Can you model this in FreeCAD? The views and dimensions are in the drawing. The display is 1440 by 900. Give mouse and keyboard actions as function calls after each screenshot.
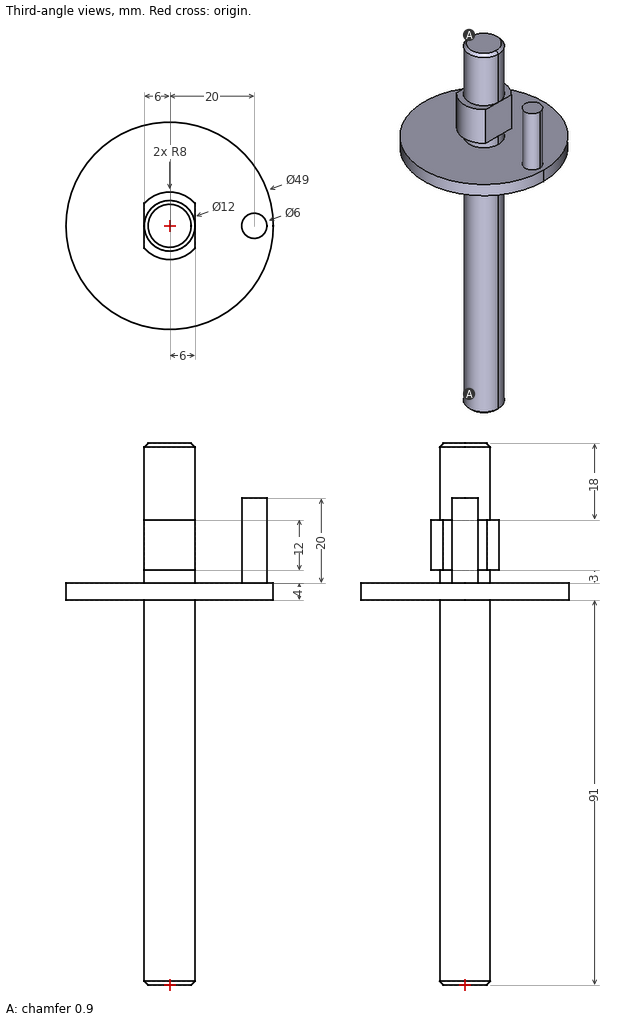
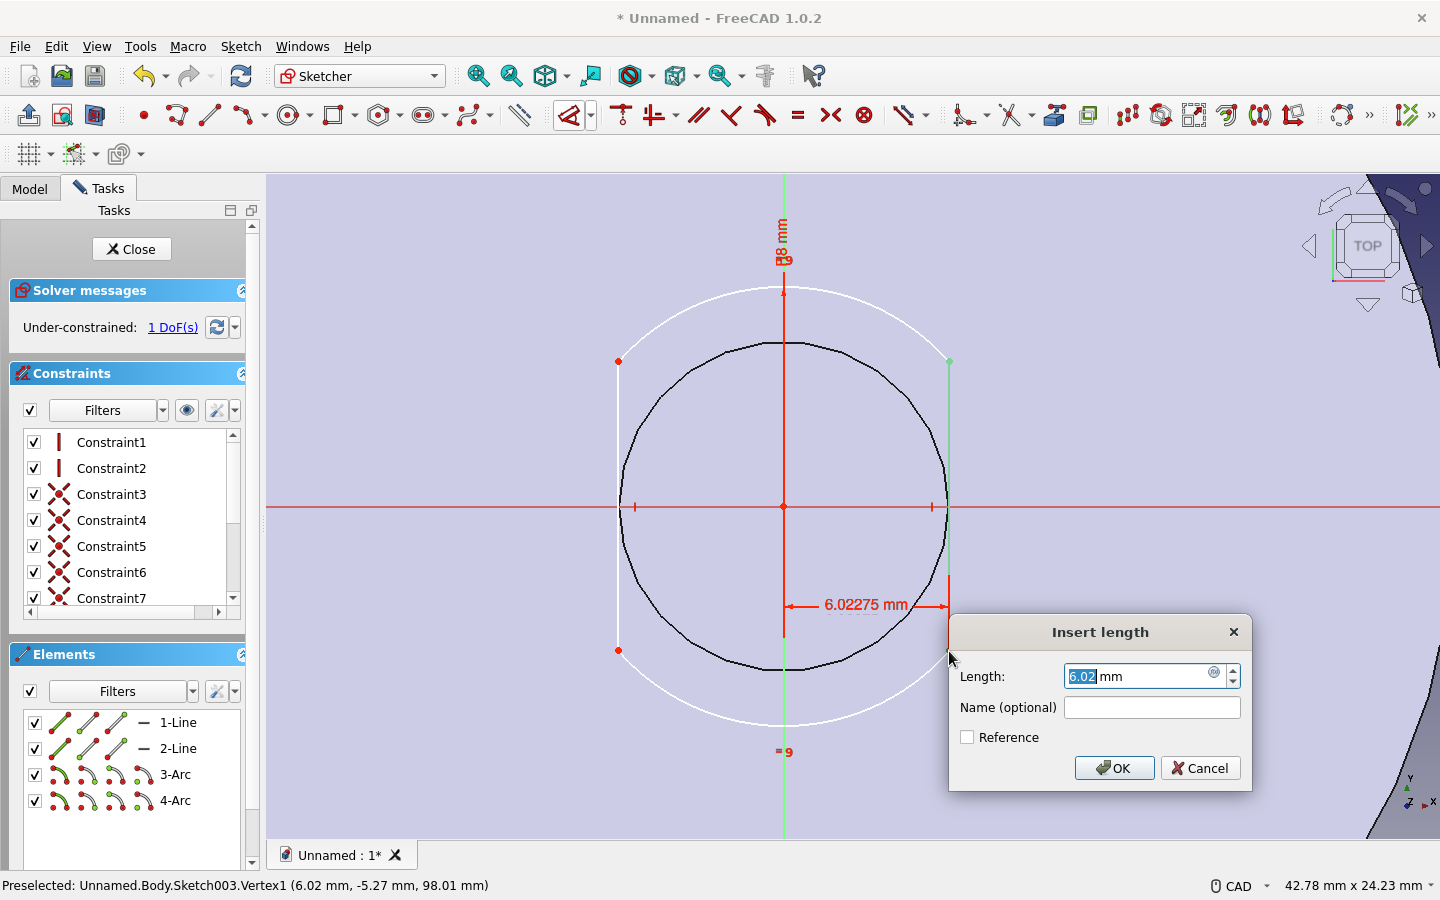
text(6)
key(Return)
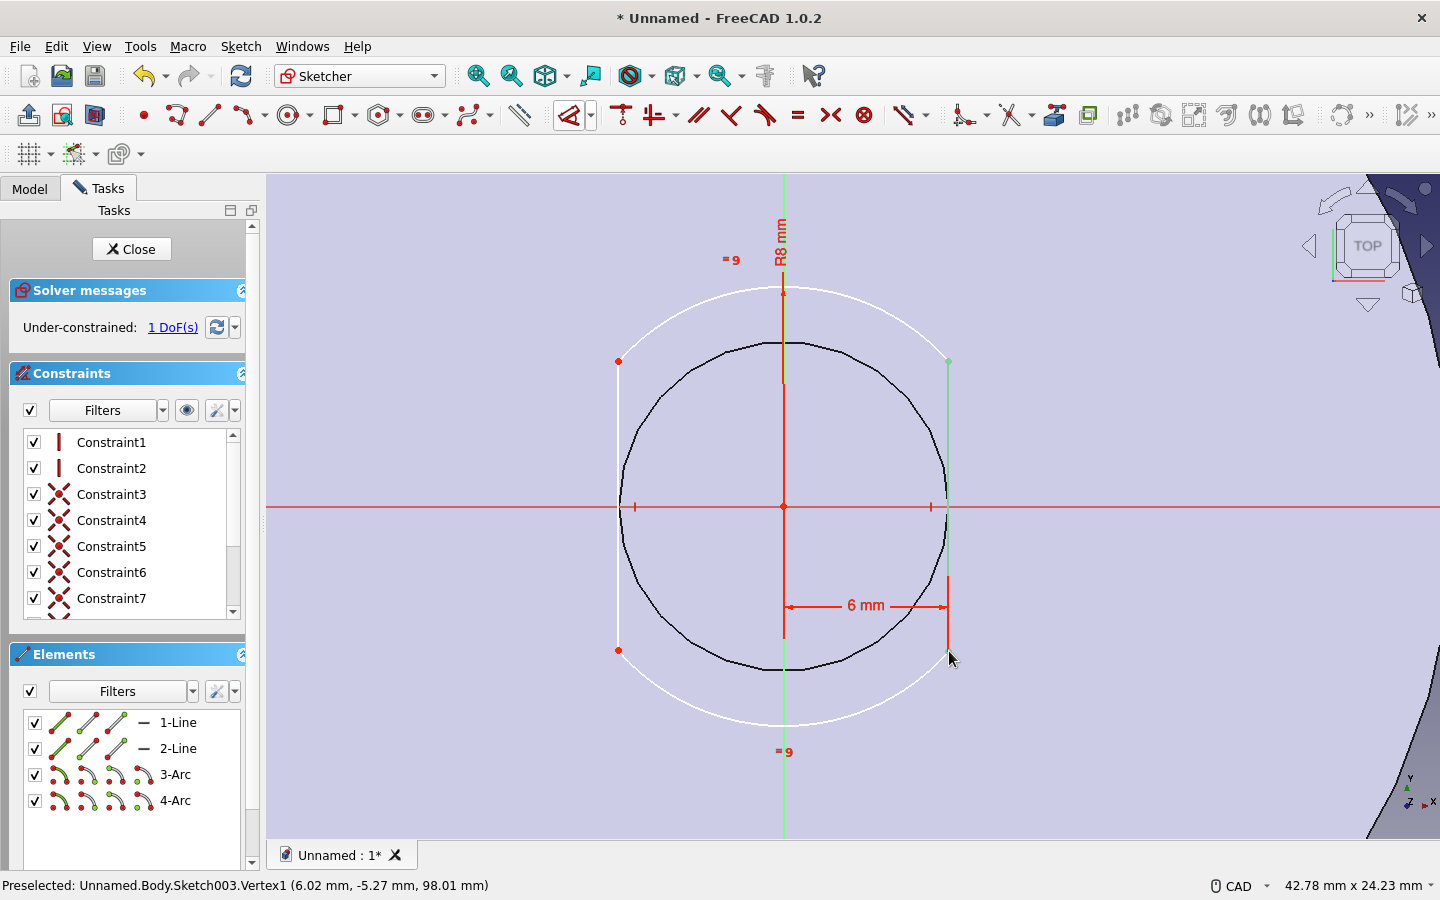
click(618, 362)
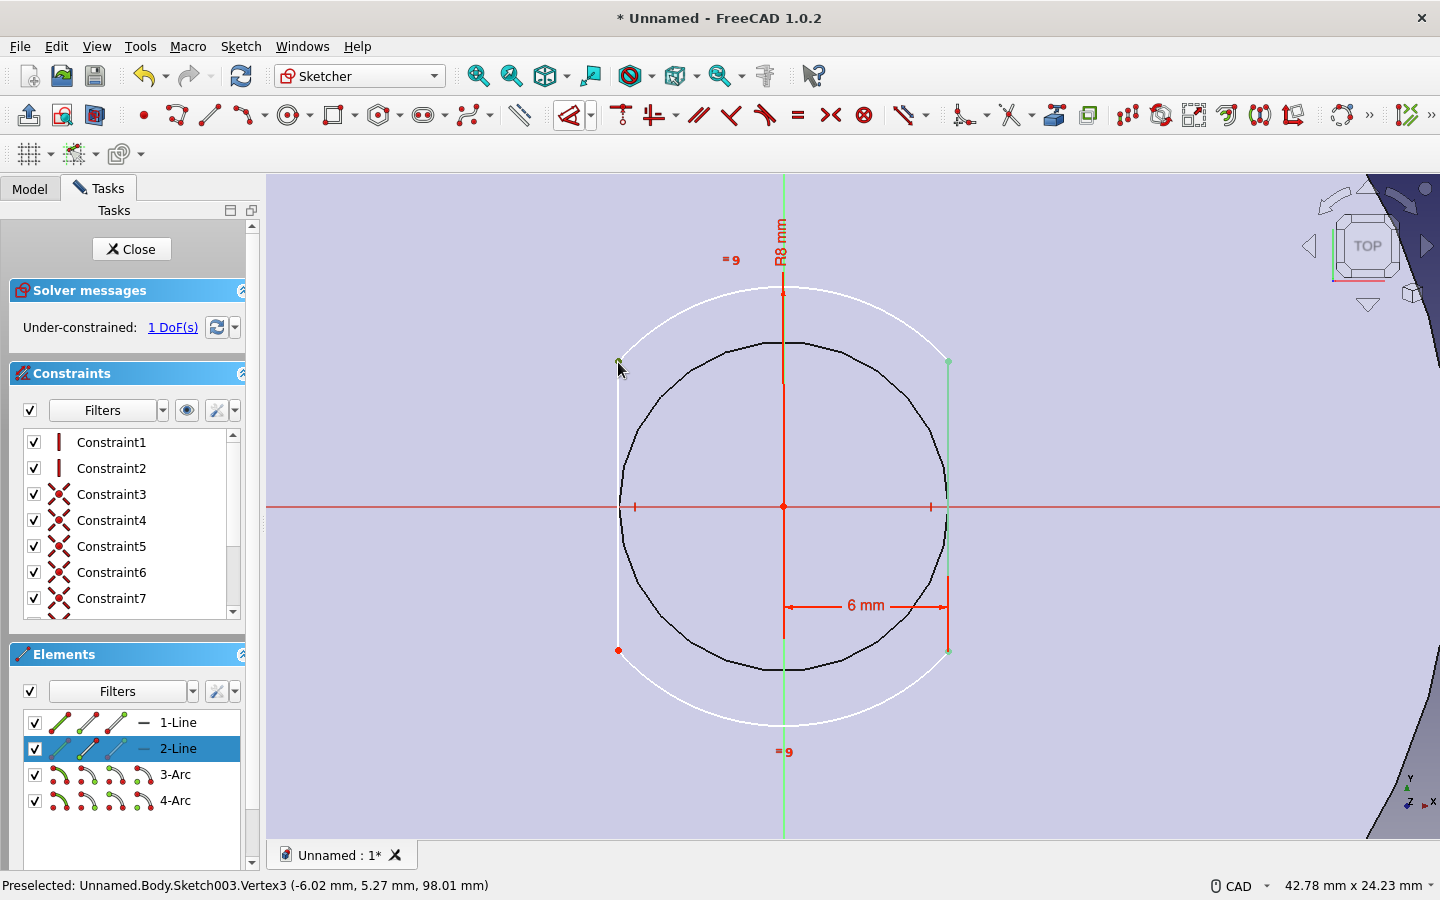
key(l)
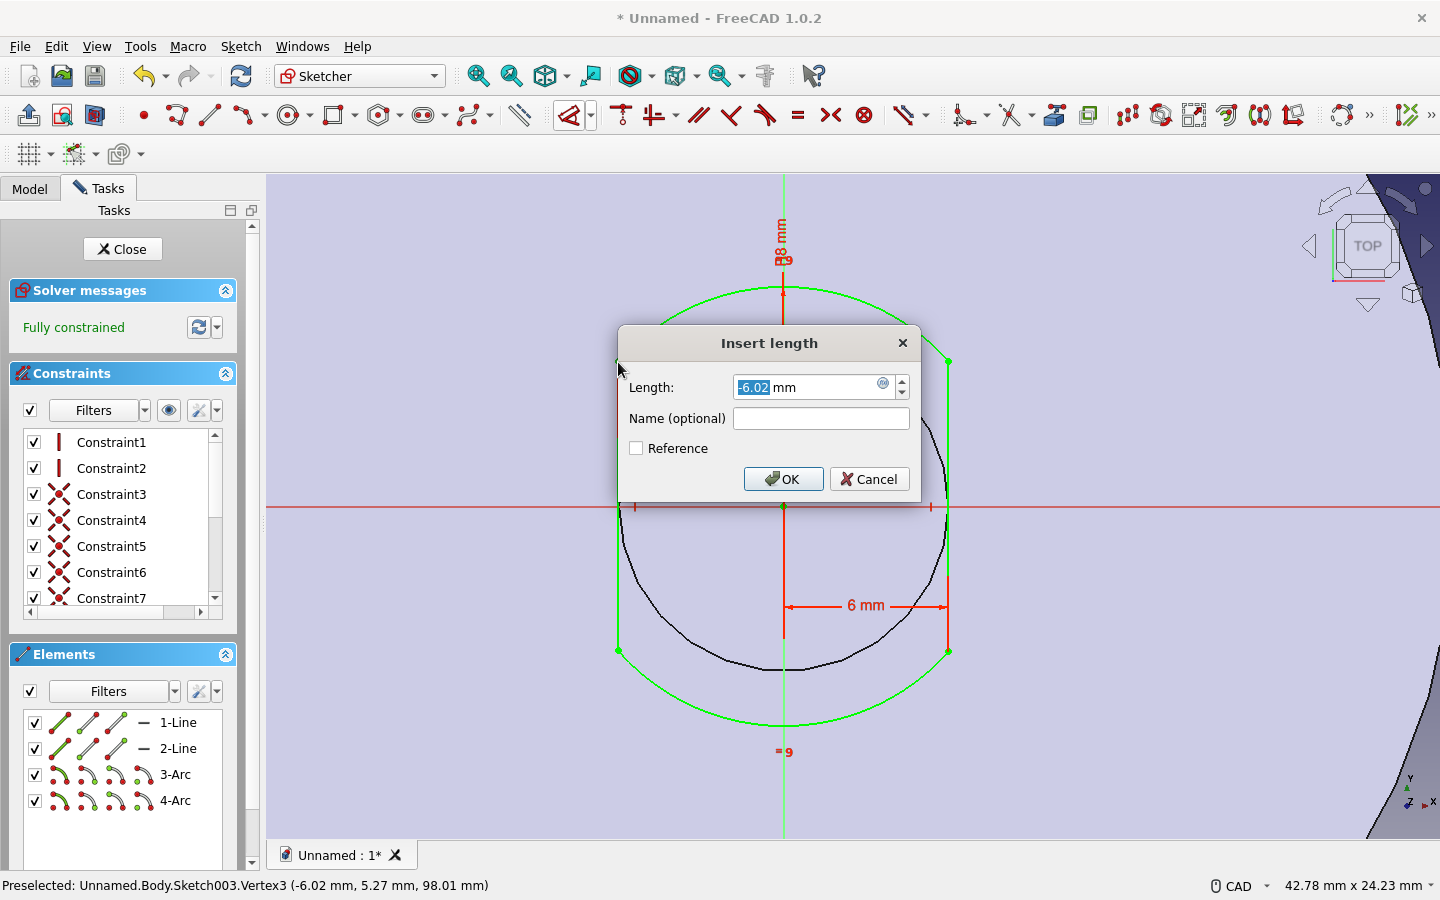
text(-6)
key(Return)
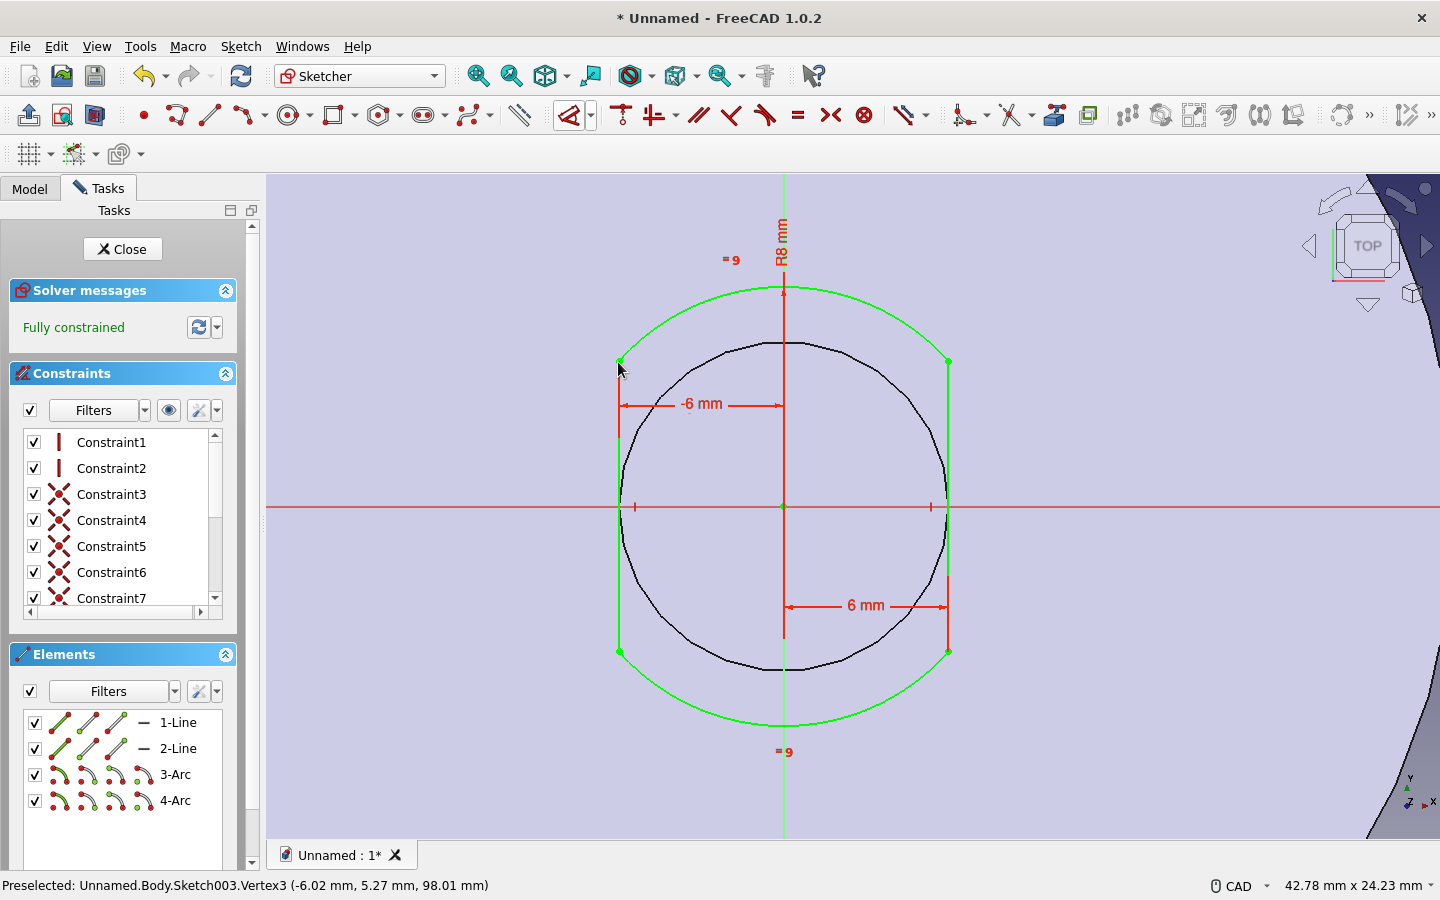
click(123, 249)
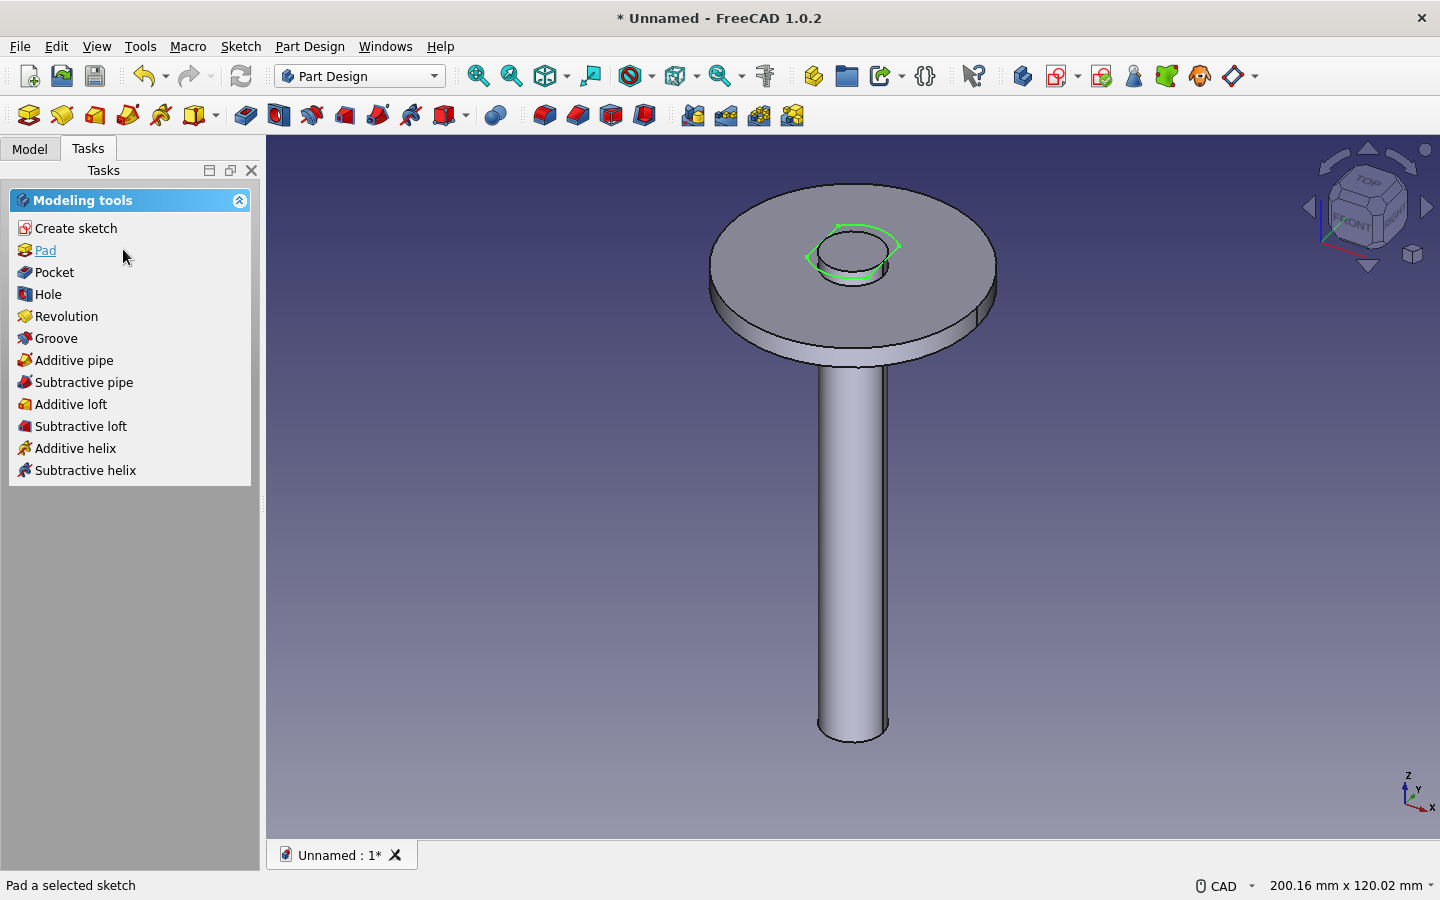
click(29, 116)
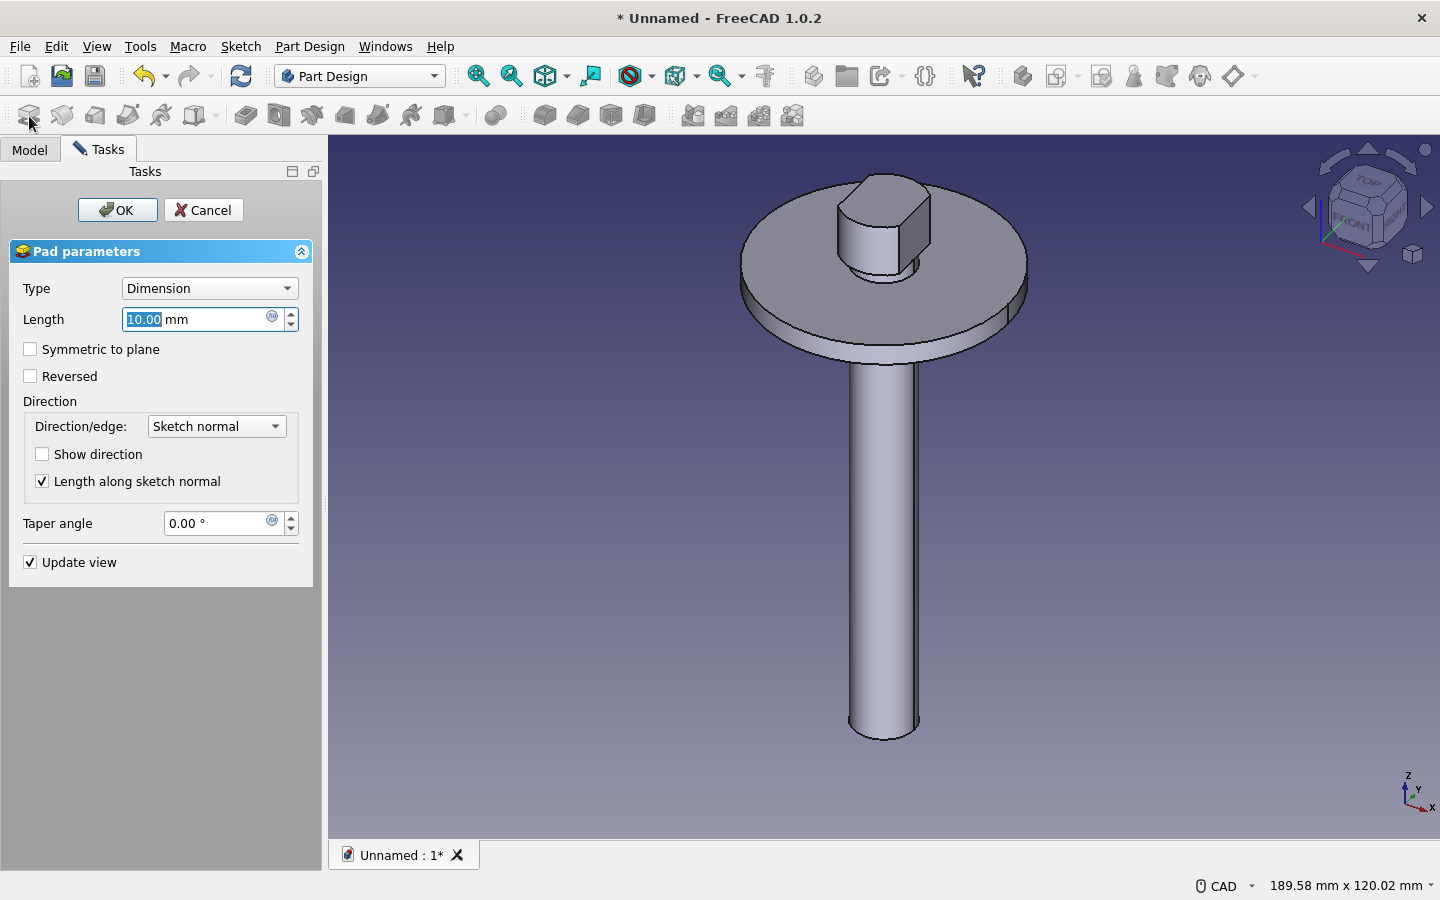
text(12)
key(Tab)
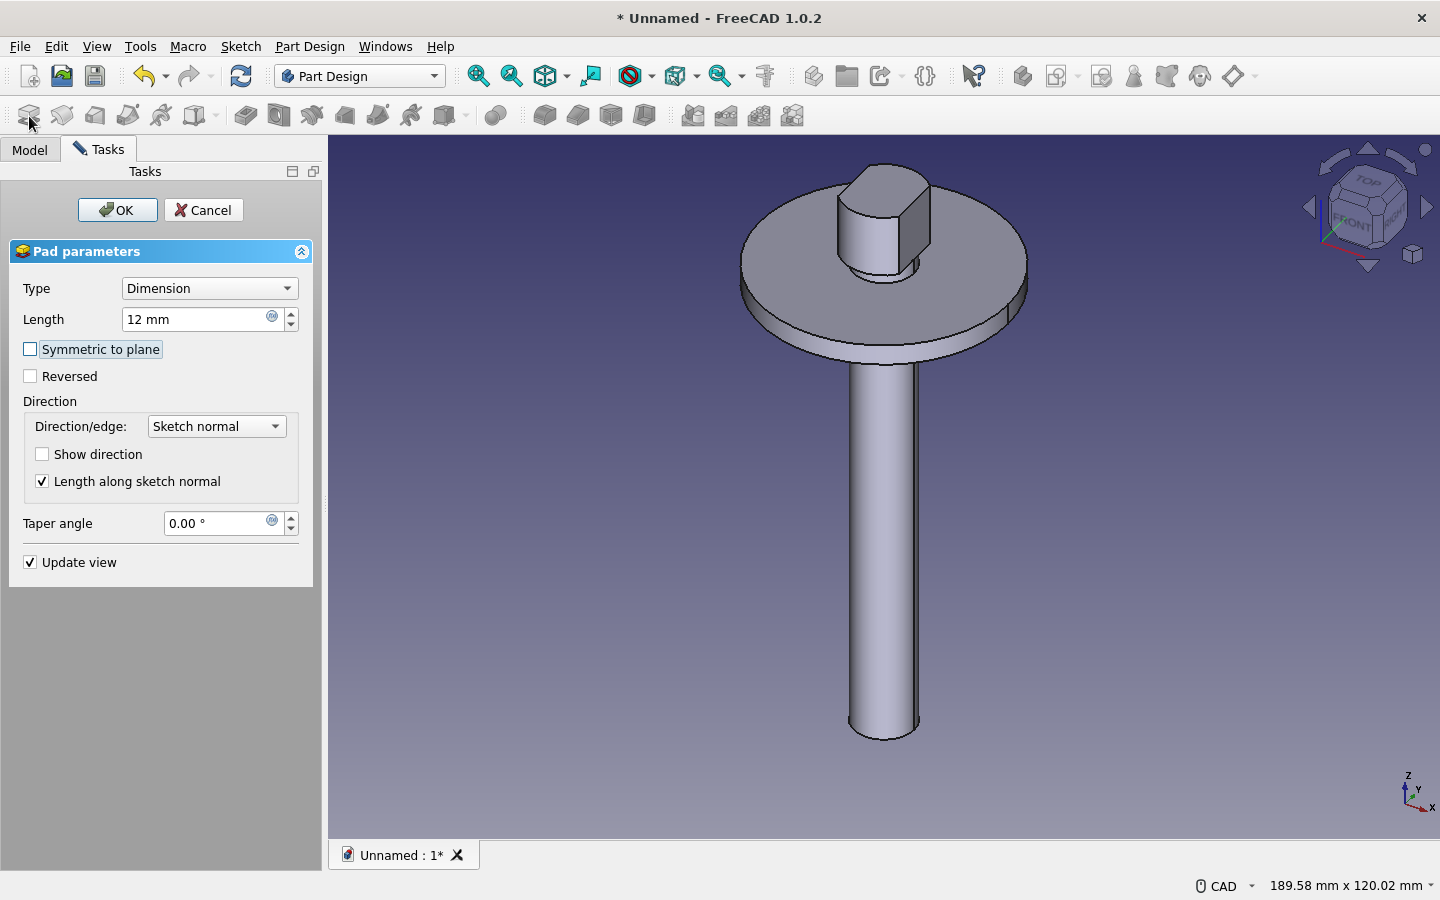
click(118, 210)